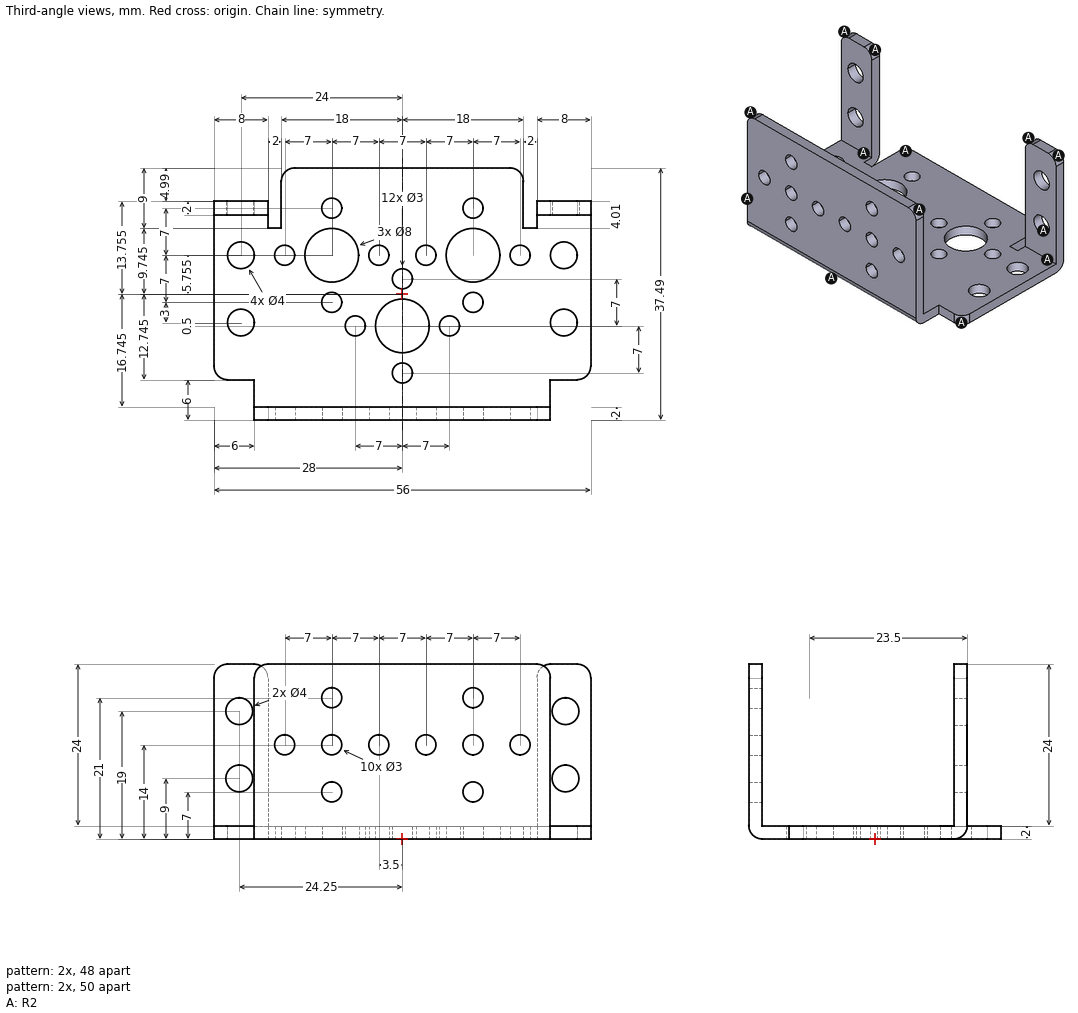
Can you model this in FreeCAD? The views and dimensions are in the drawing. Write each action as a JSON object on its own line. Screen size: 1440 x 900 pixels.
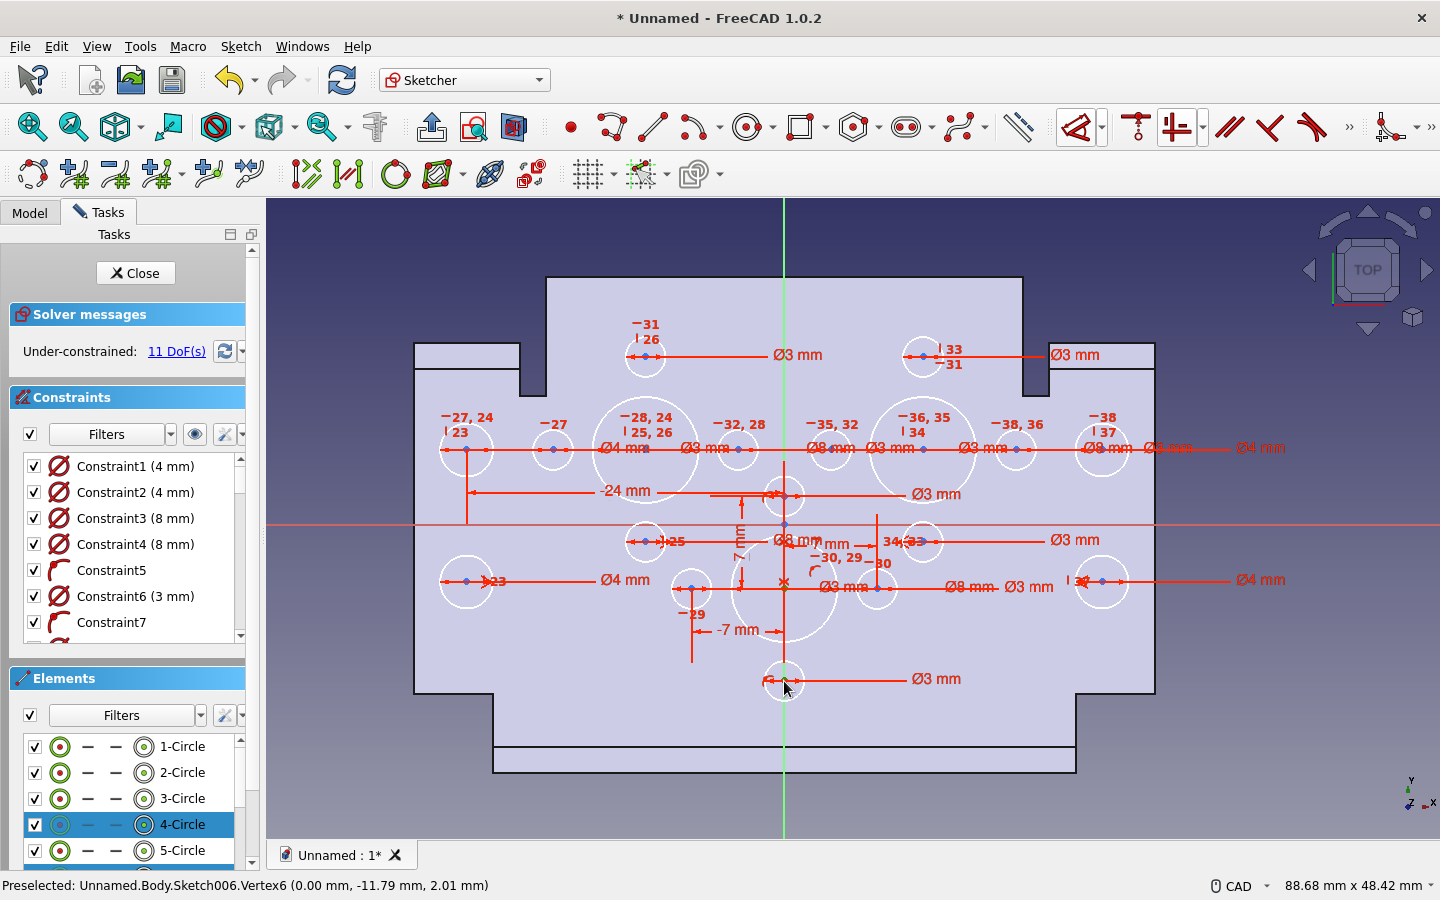
{"action": "left_click", "coordinate": [1102, 128]}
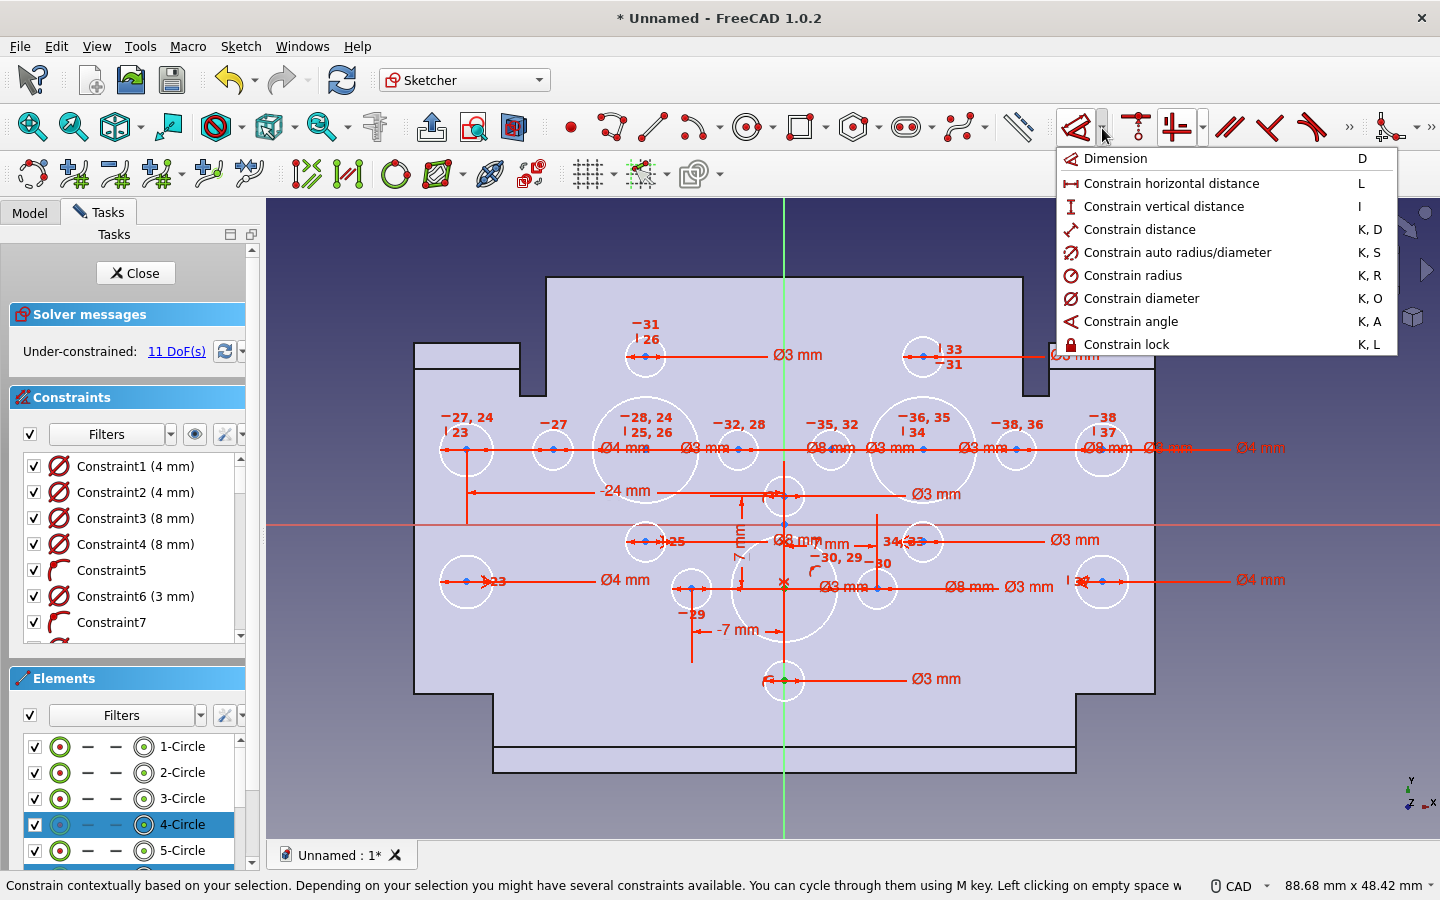
{"action": "left_click", "coordinate": [1227, 206]}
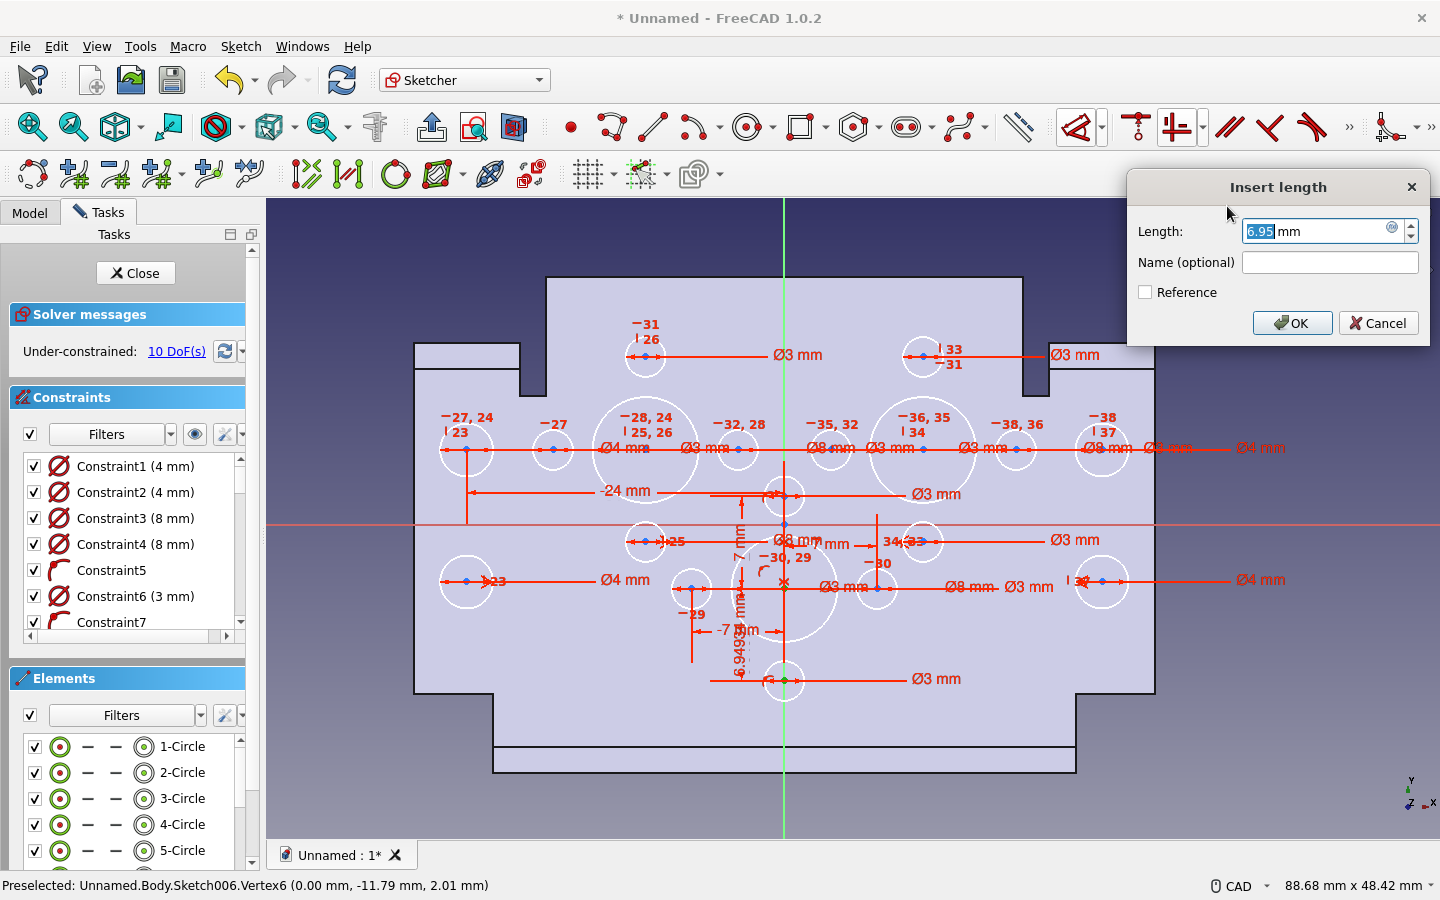
{"action": "type", "text": "7"}
{"action": "key", "text": "Return"}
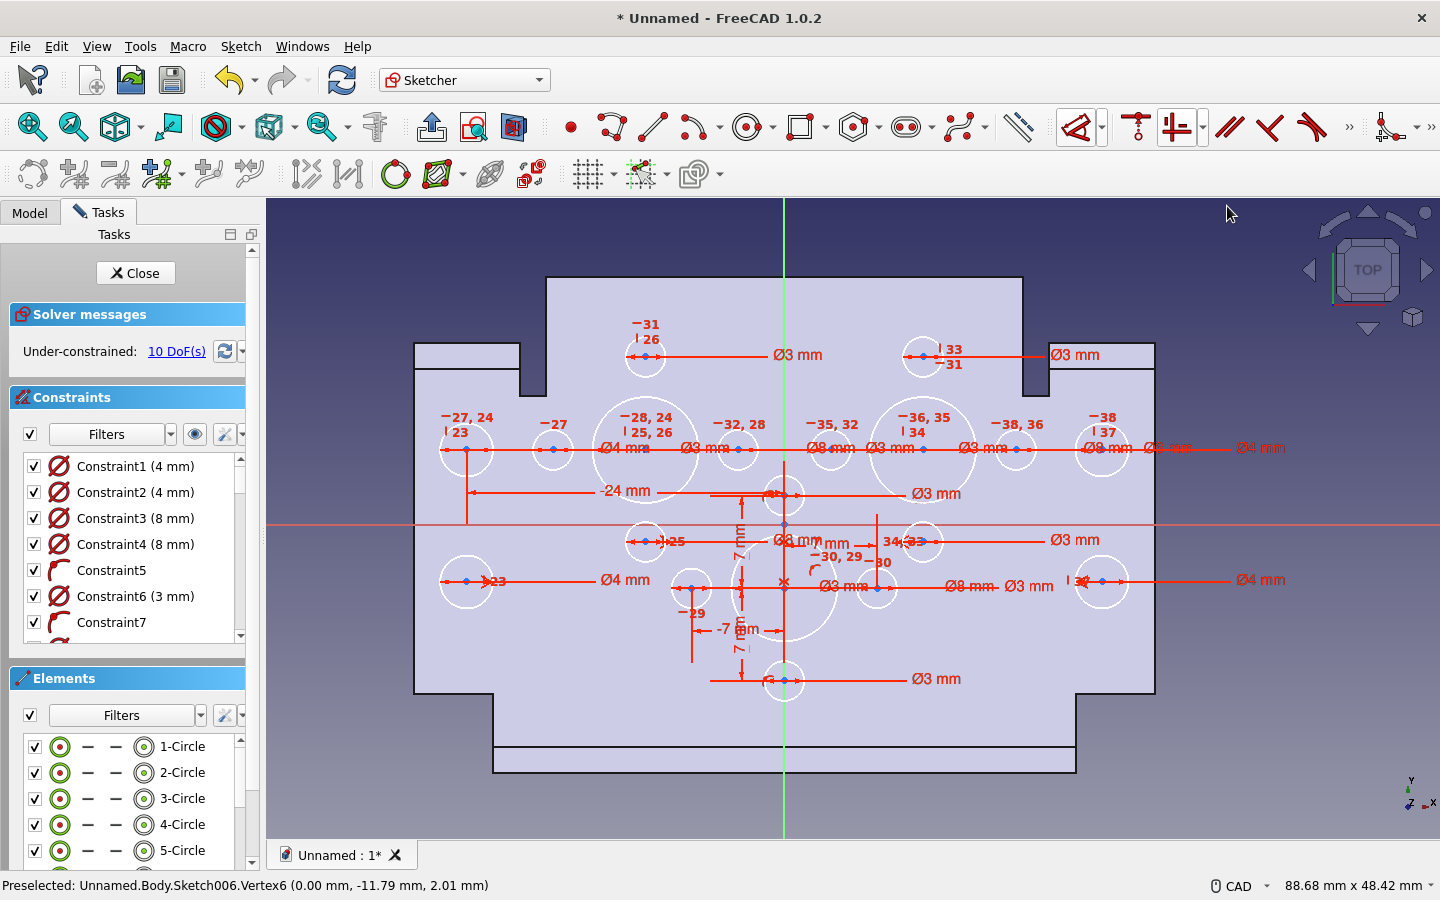
{"action": "left_click", "coordinate": [646, 450]}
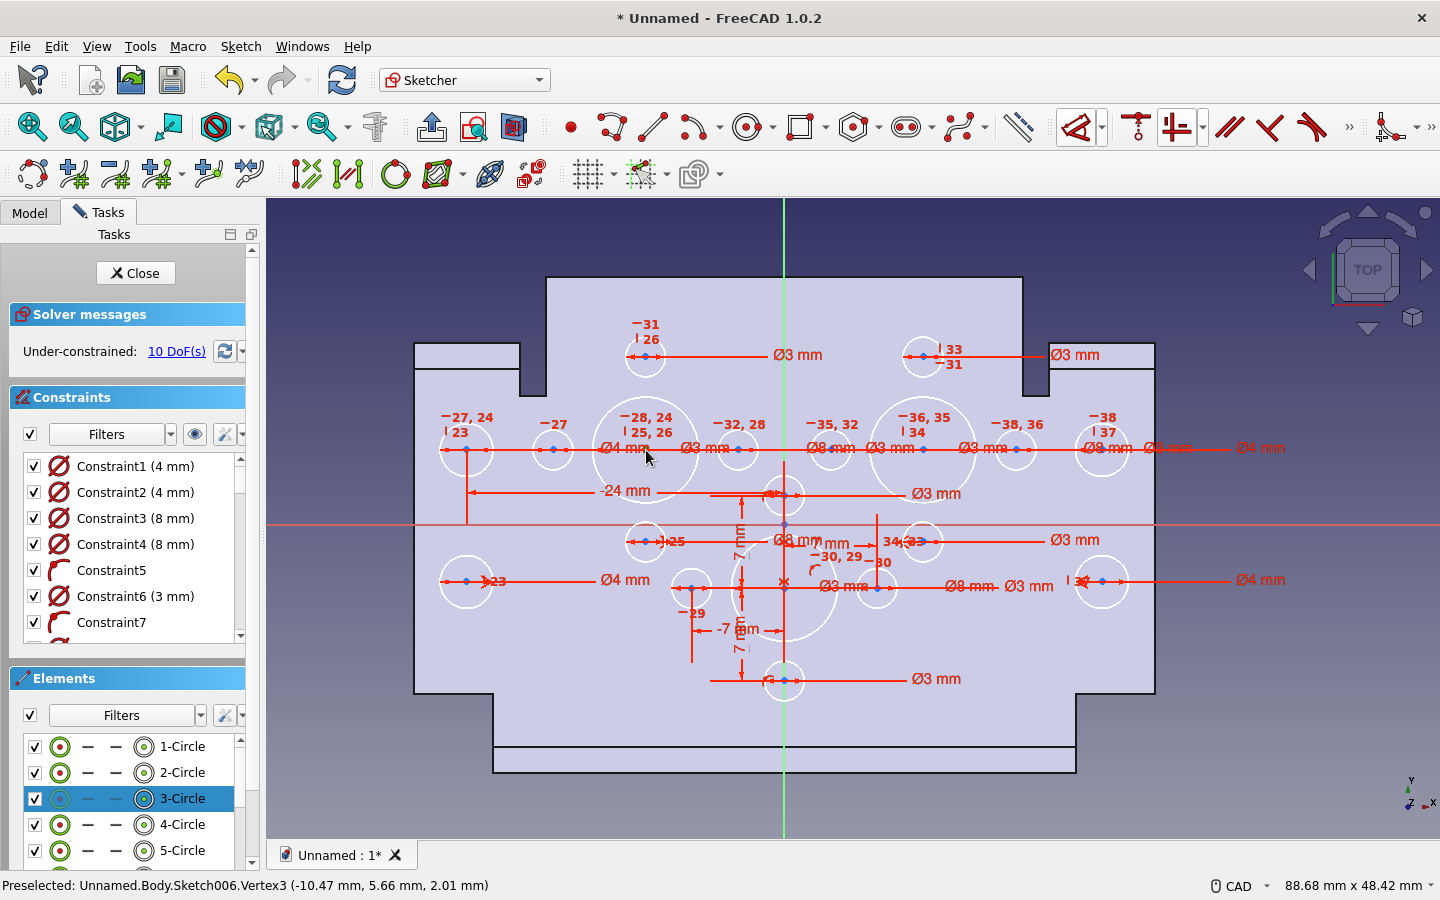
{"action": "left_click", "coordinate": [646, 542]}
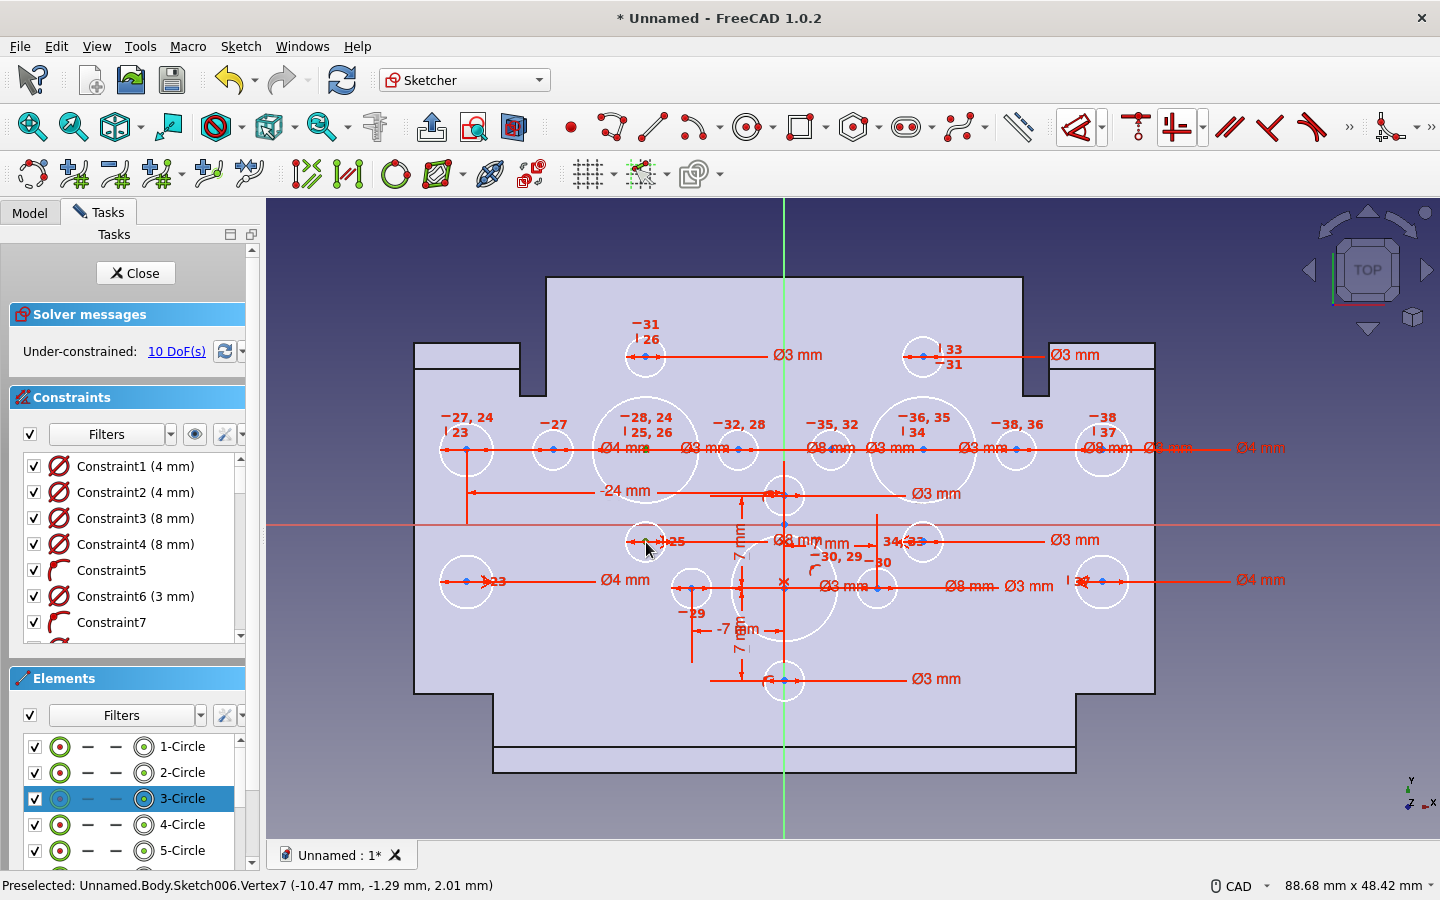
{"action": "left_click", "coordinate": [1102, 128]}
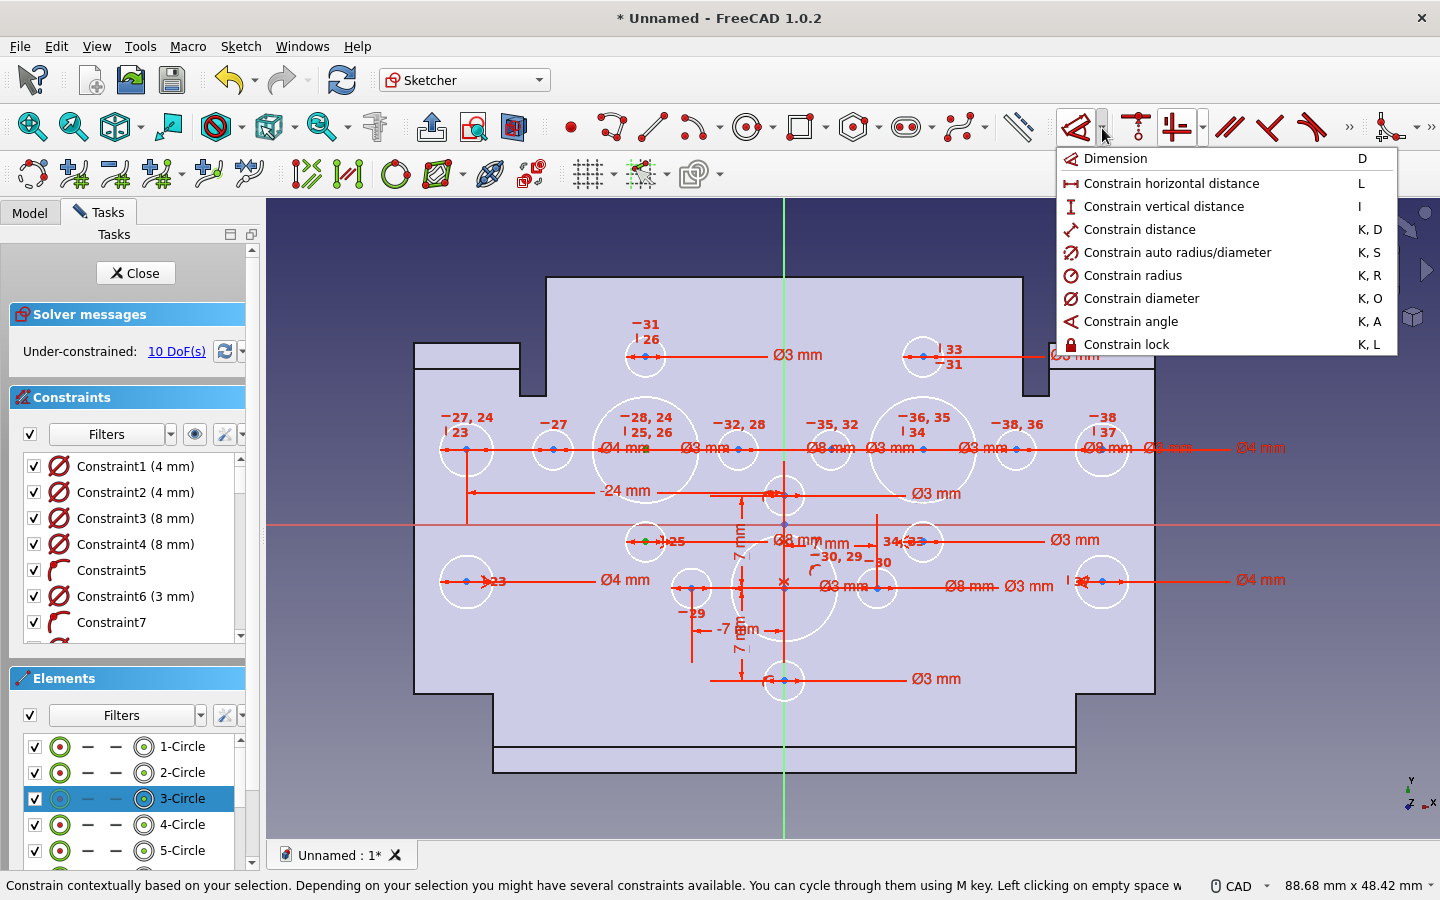
{"action": "left_click", "coordinate": [1227, 206]}